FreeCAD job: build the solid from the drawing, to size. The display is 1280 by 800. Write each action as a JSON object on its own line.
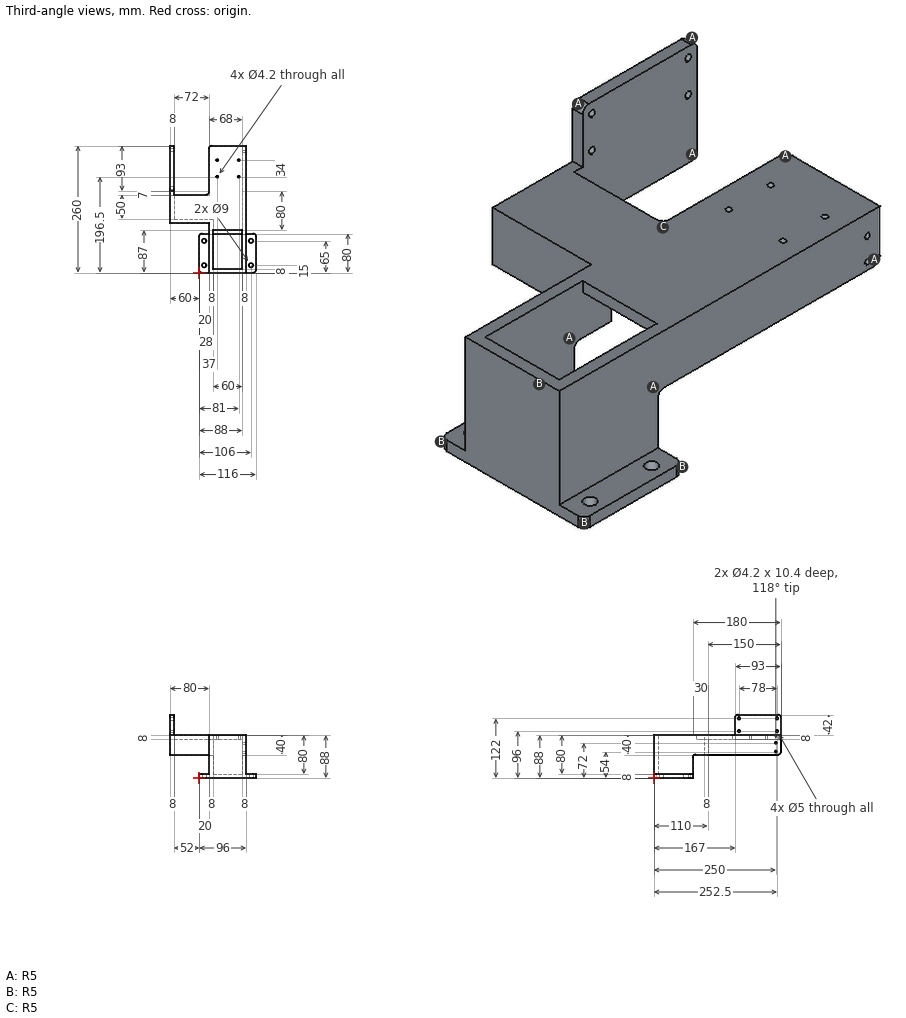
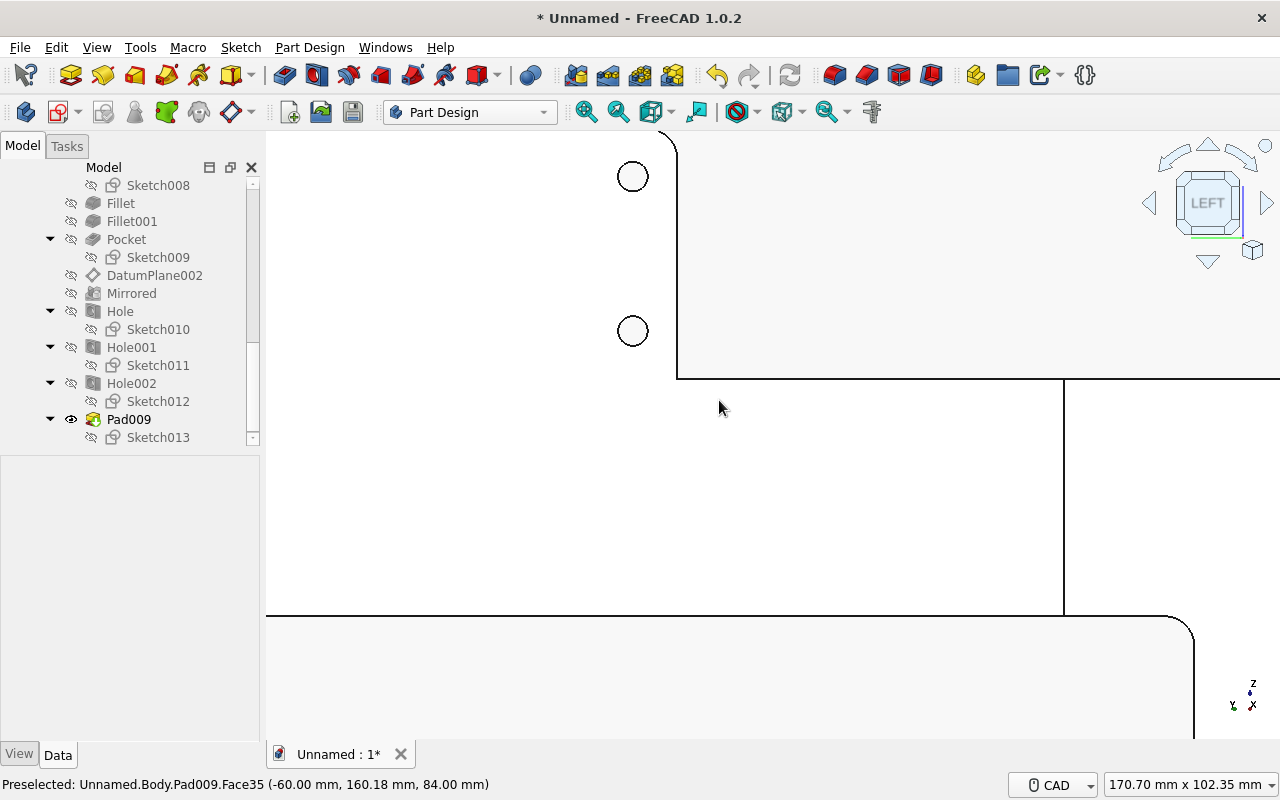
{"action": "left_click", "coordinate": [588, 112]}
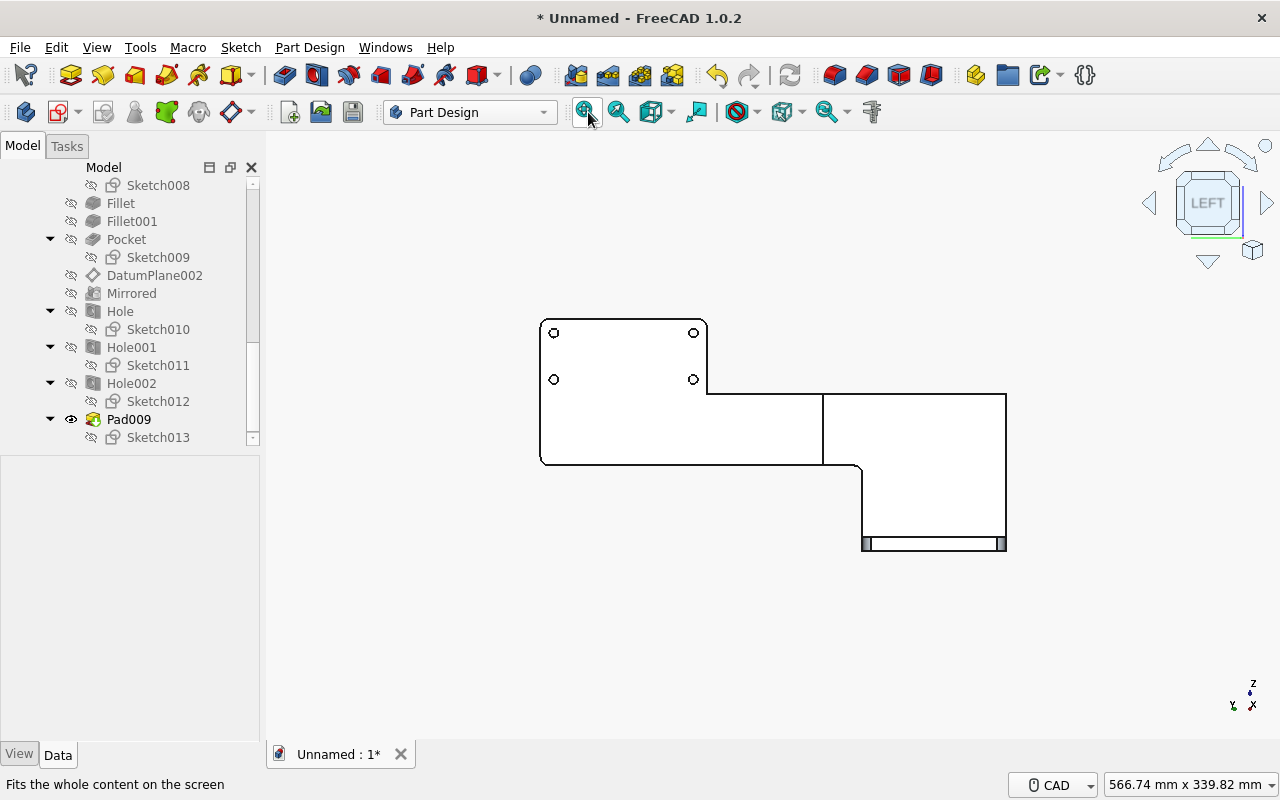
{"action": "key", "text": "v 3"}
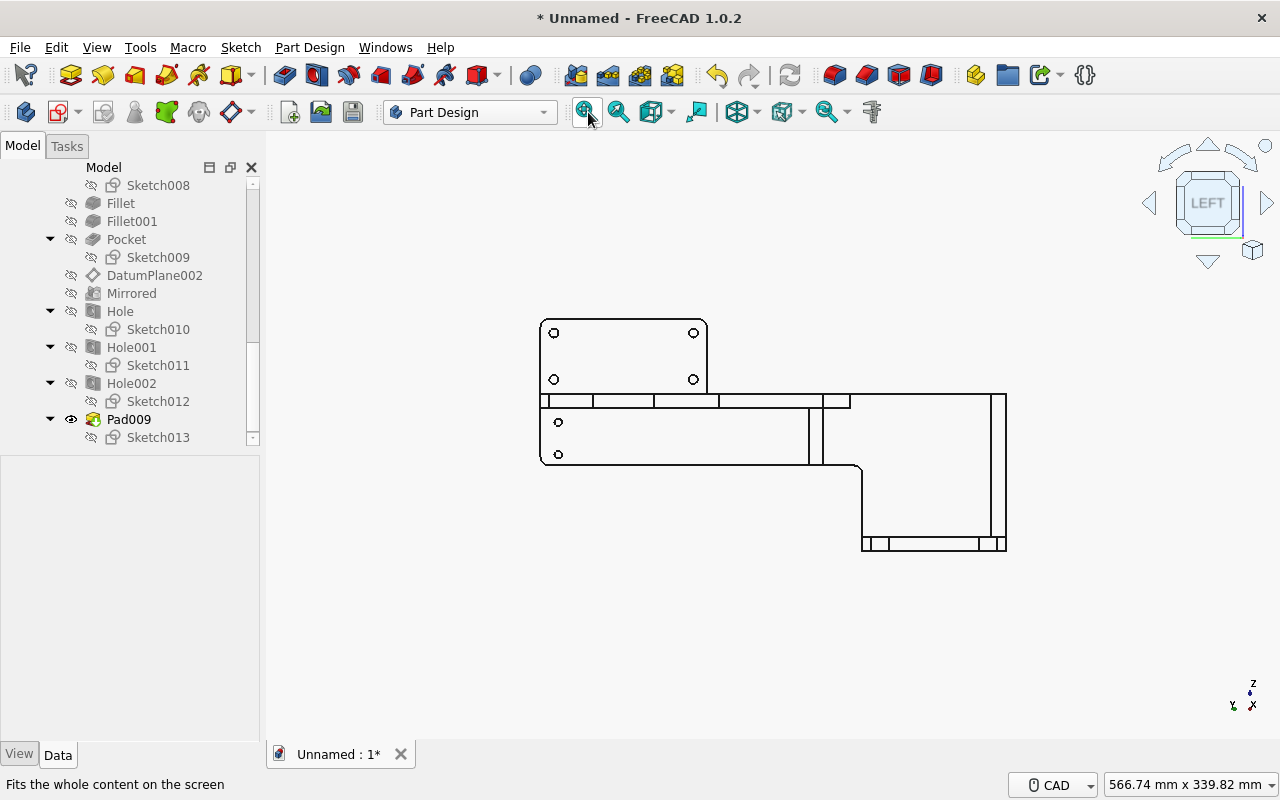
{"action": "key", "text": "0"}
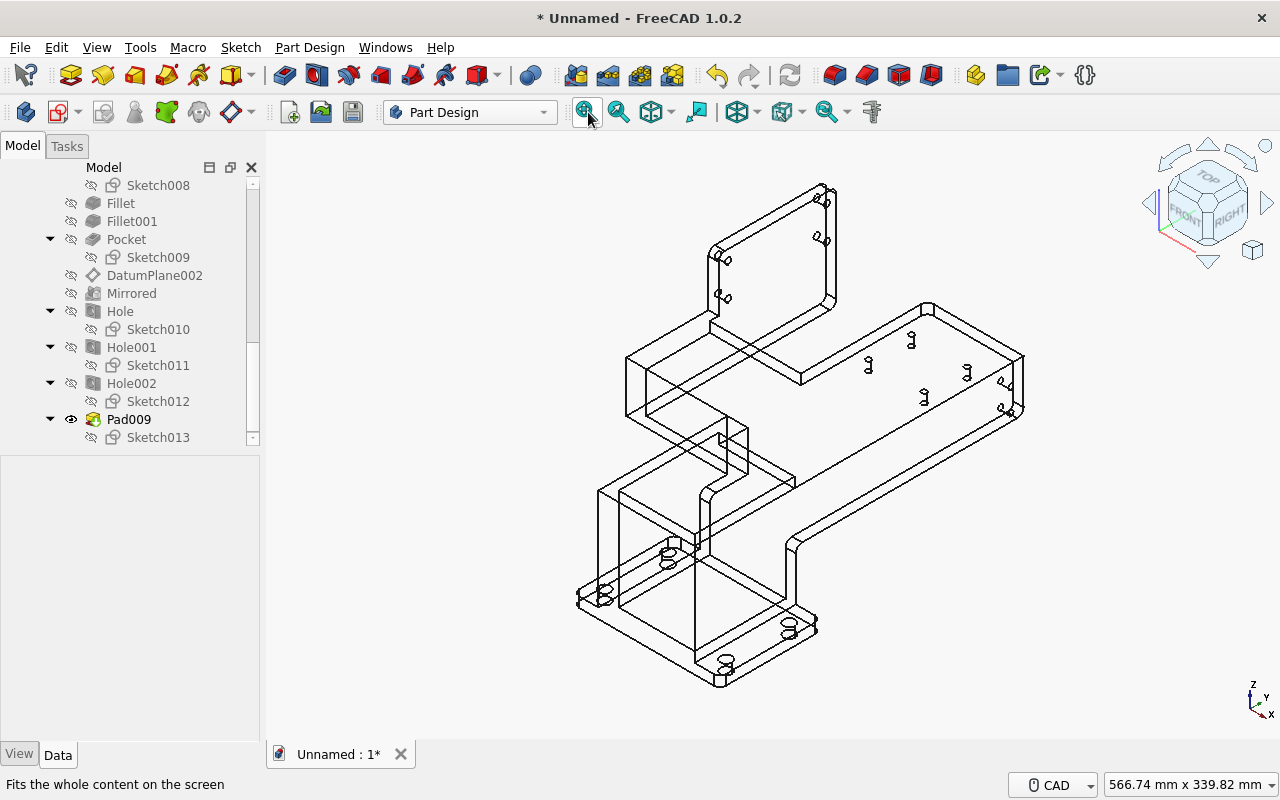
{"action": "left_click", "coordinate": [801, 380]}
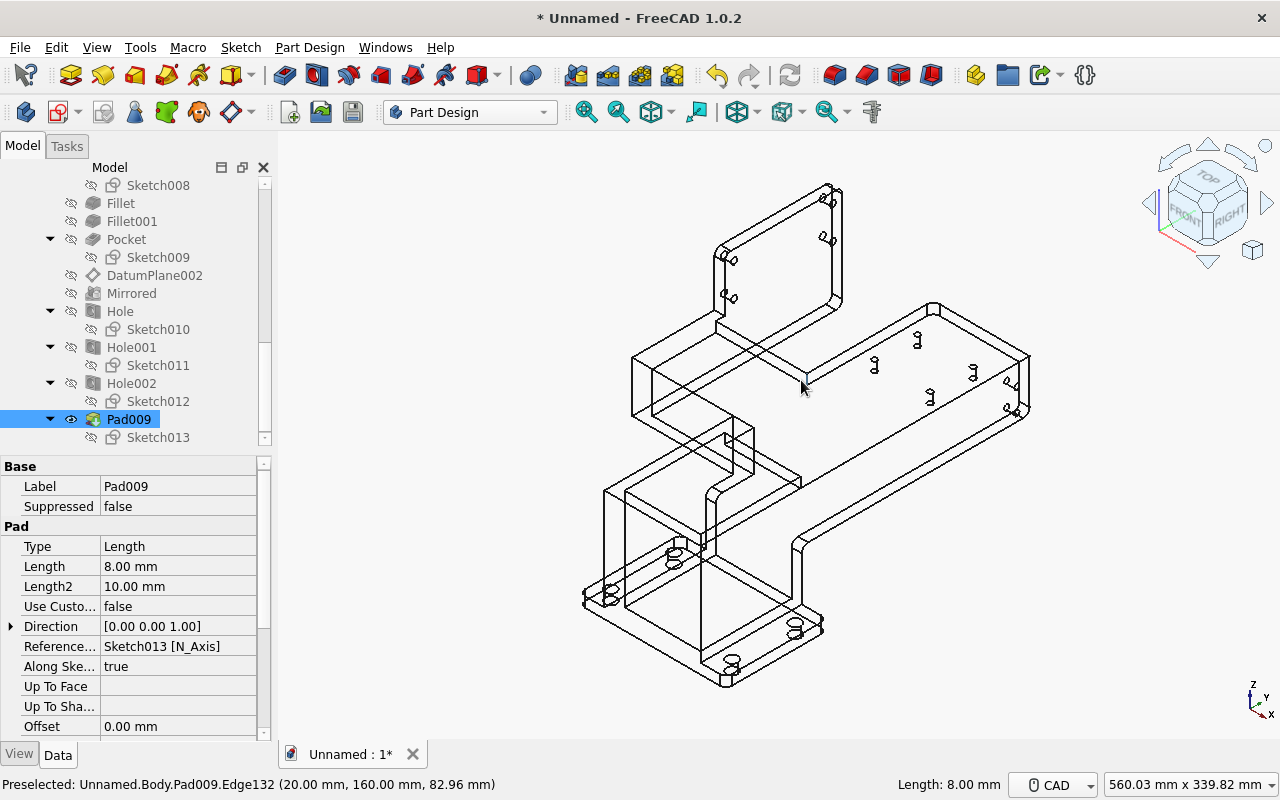
{"action": "key", "text": "v 1"}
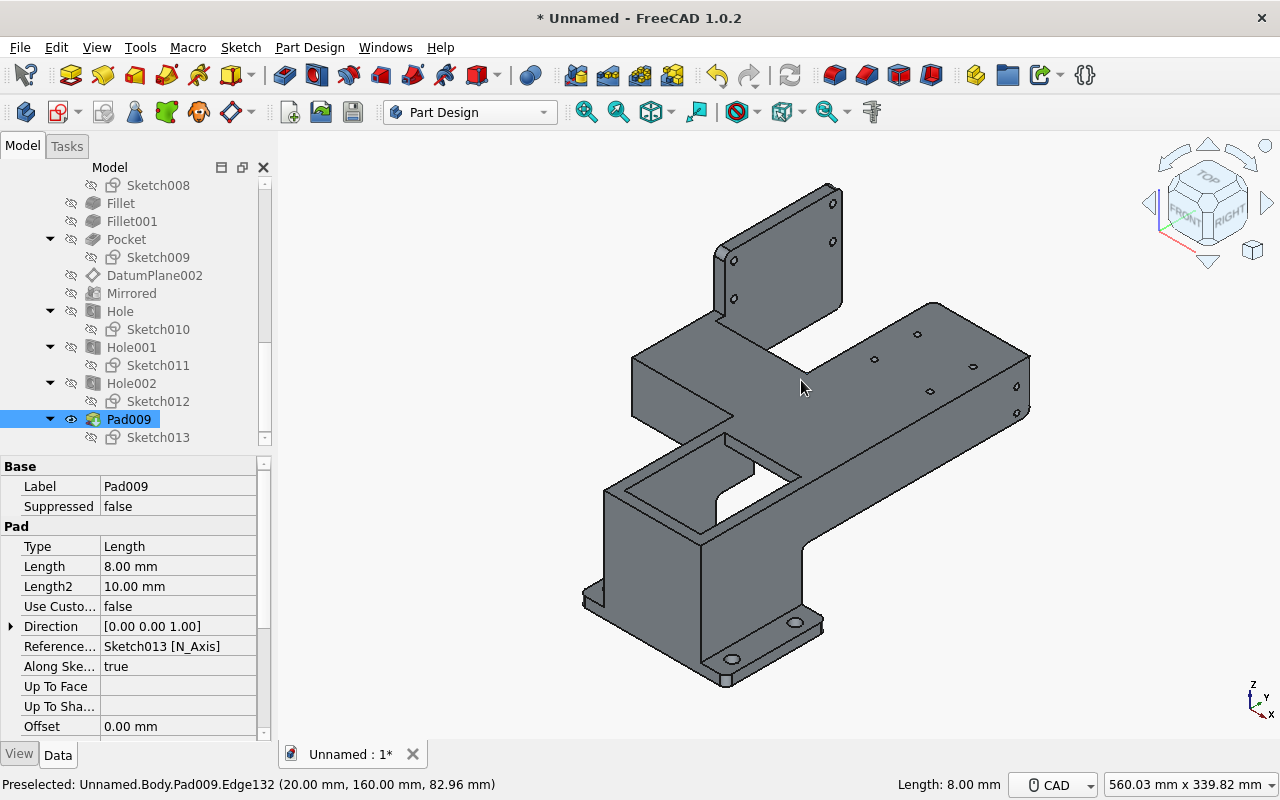
{"action": "left_click", "coordinate": [836, 76]}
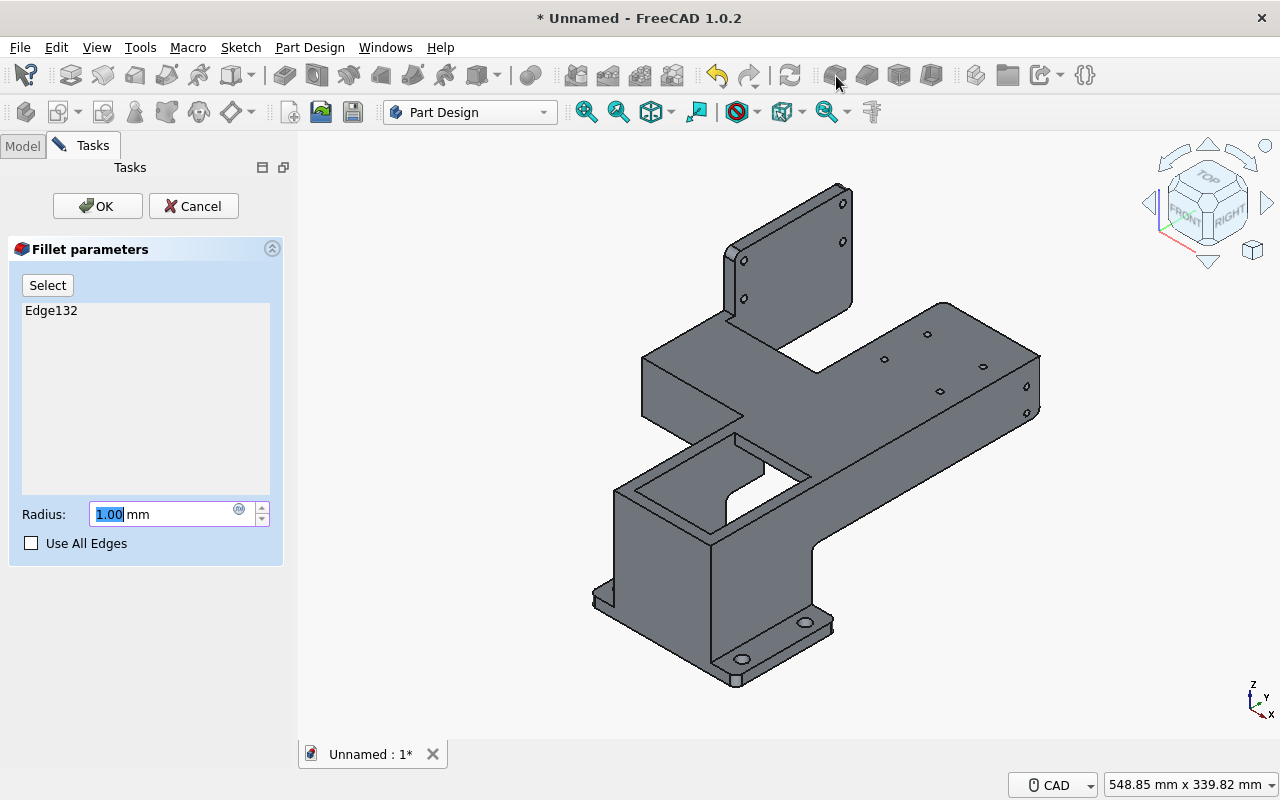
{"action": "type", "text": "5"}
{"action": "key", "text": "Tab"}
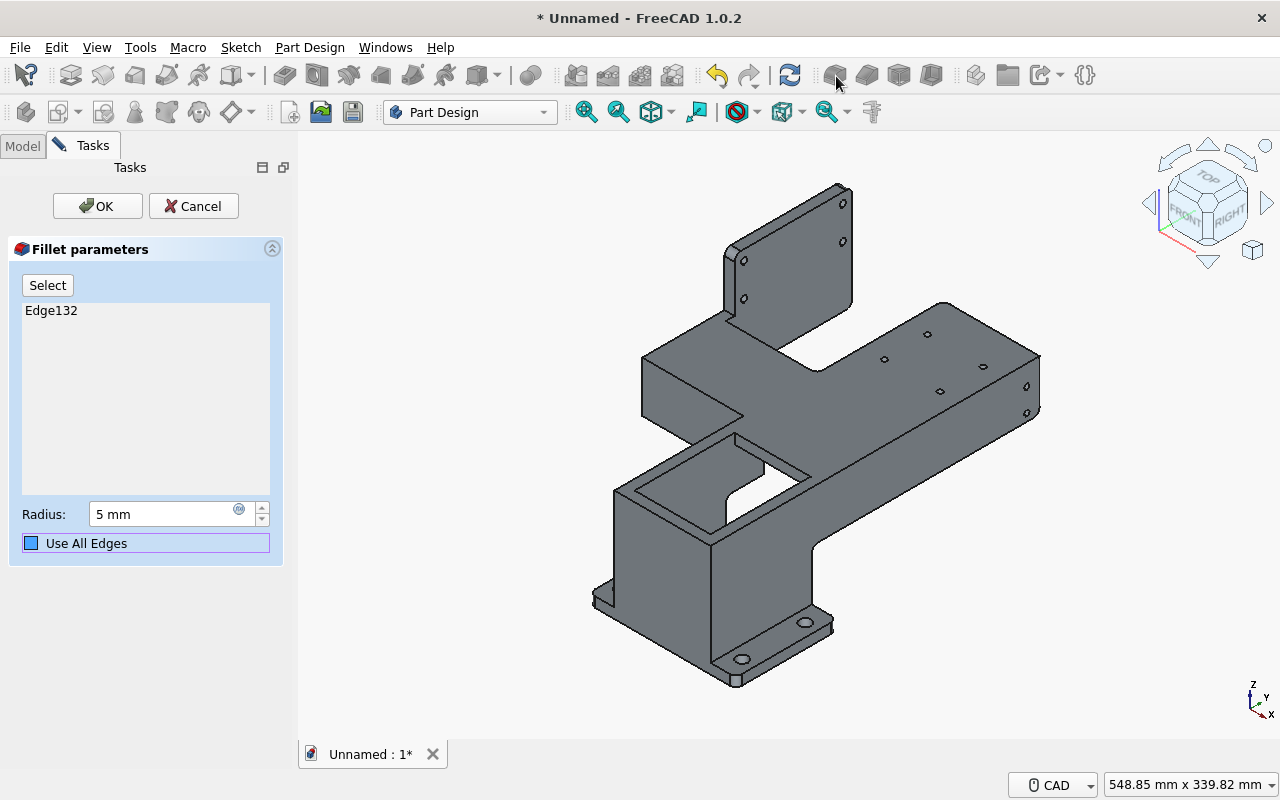
{"action": "left_click", "coordinate": [98, 206]}